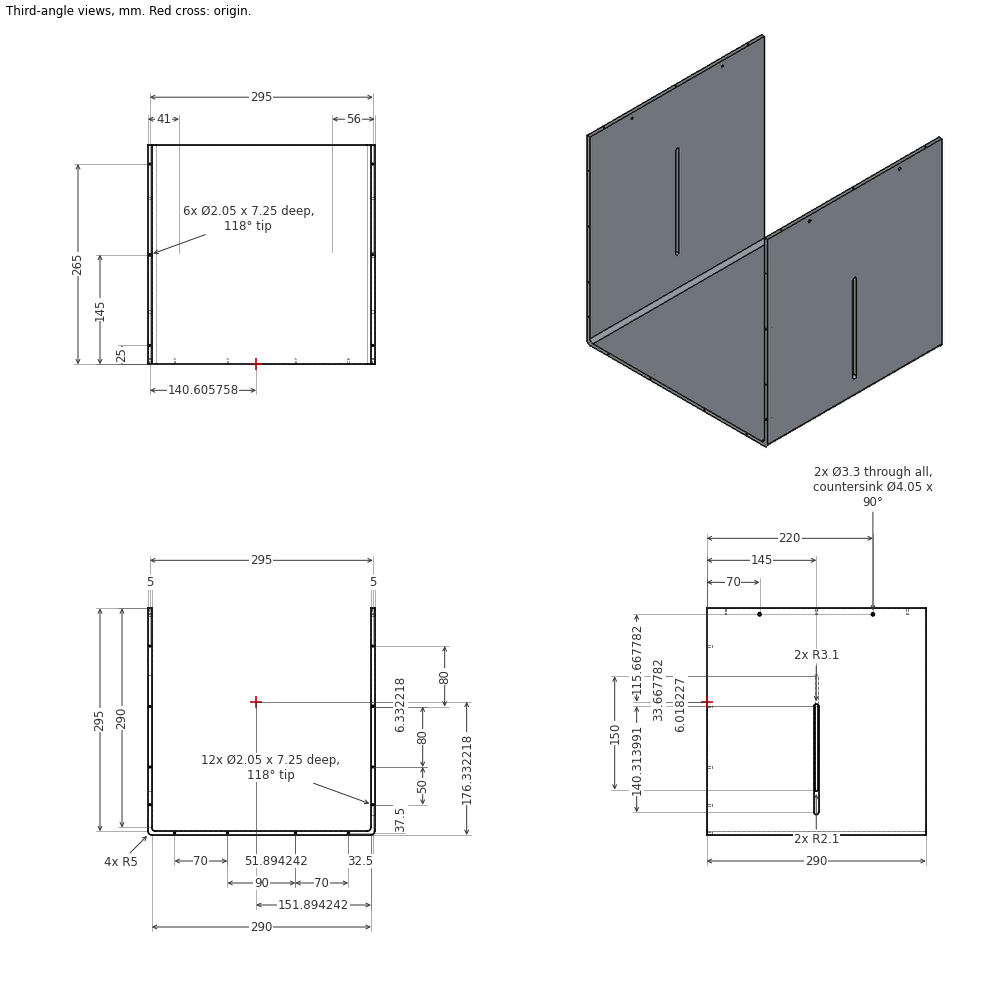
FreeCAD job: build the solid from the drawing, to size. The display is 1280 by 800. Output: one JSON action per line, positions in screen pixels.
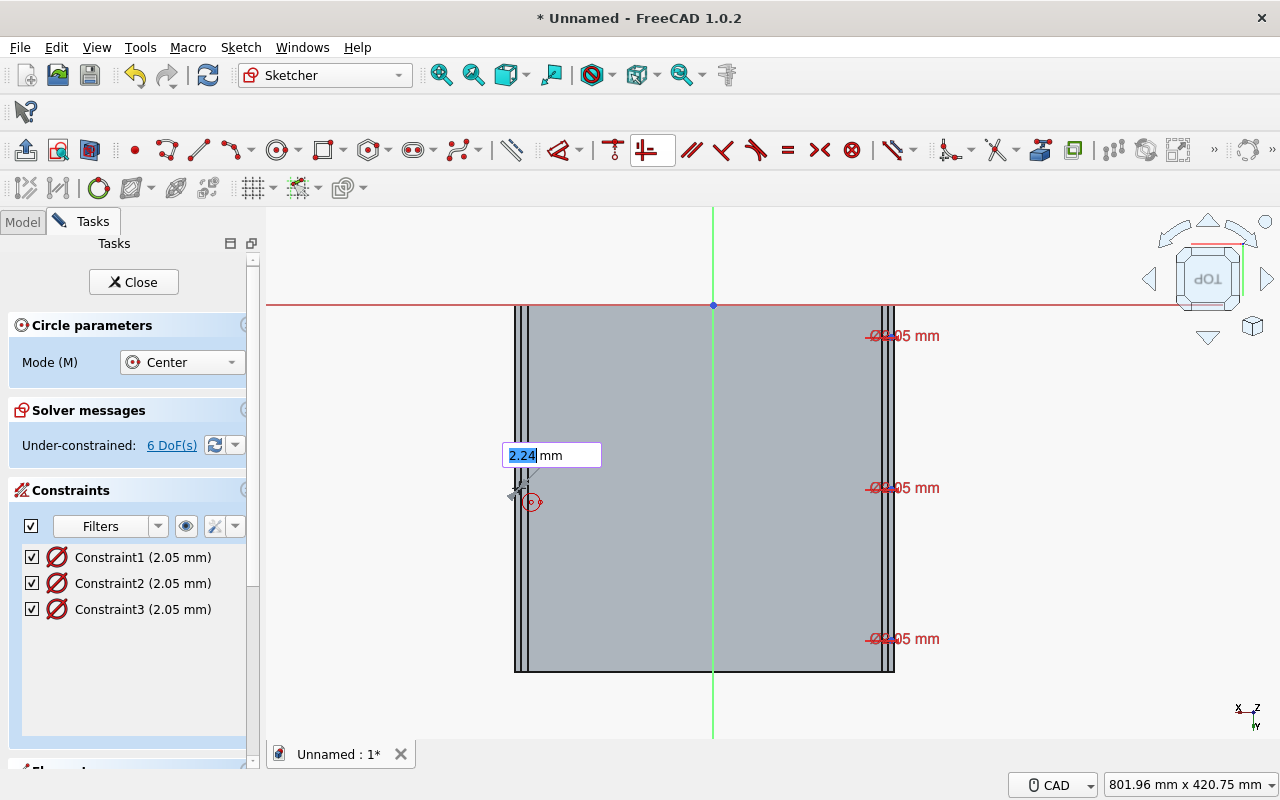
{"action": "type", "text": "2.05"}
{"action": "key", "text": "Return"}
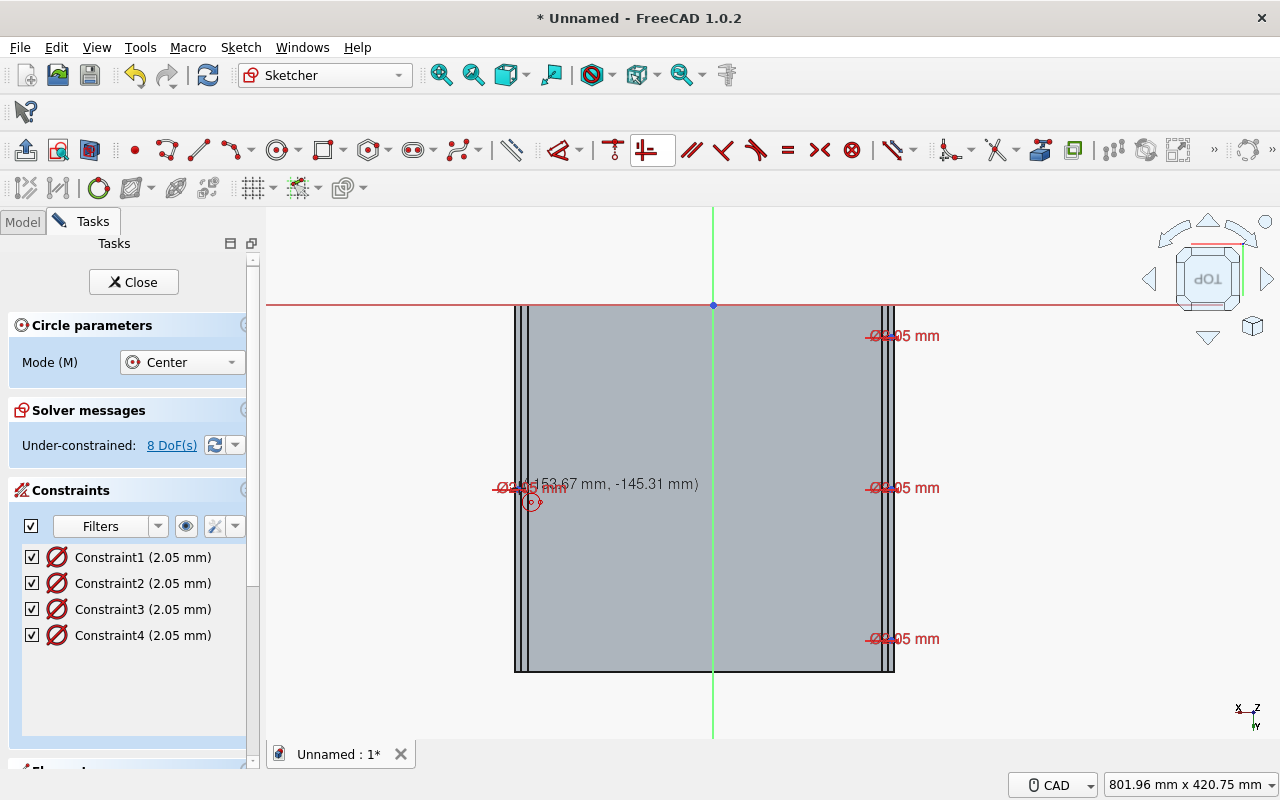
{"action": "scroll", "coordinate": [518, 640], "scroll_direction": "up", "scroll_amount": 15}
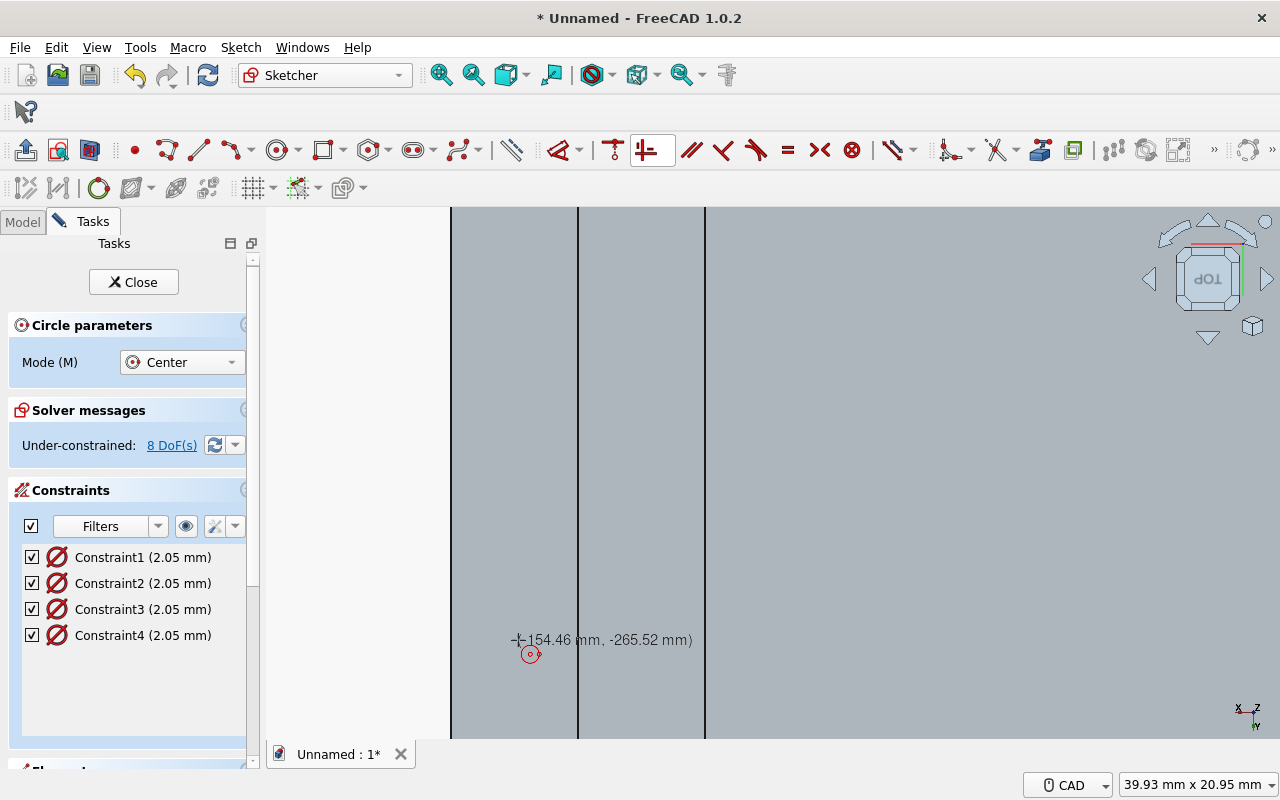
{"action": "scroll", "coordinate": [518, 640], "scroll_direction": "down", "scroll_amount": 15}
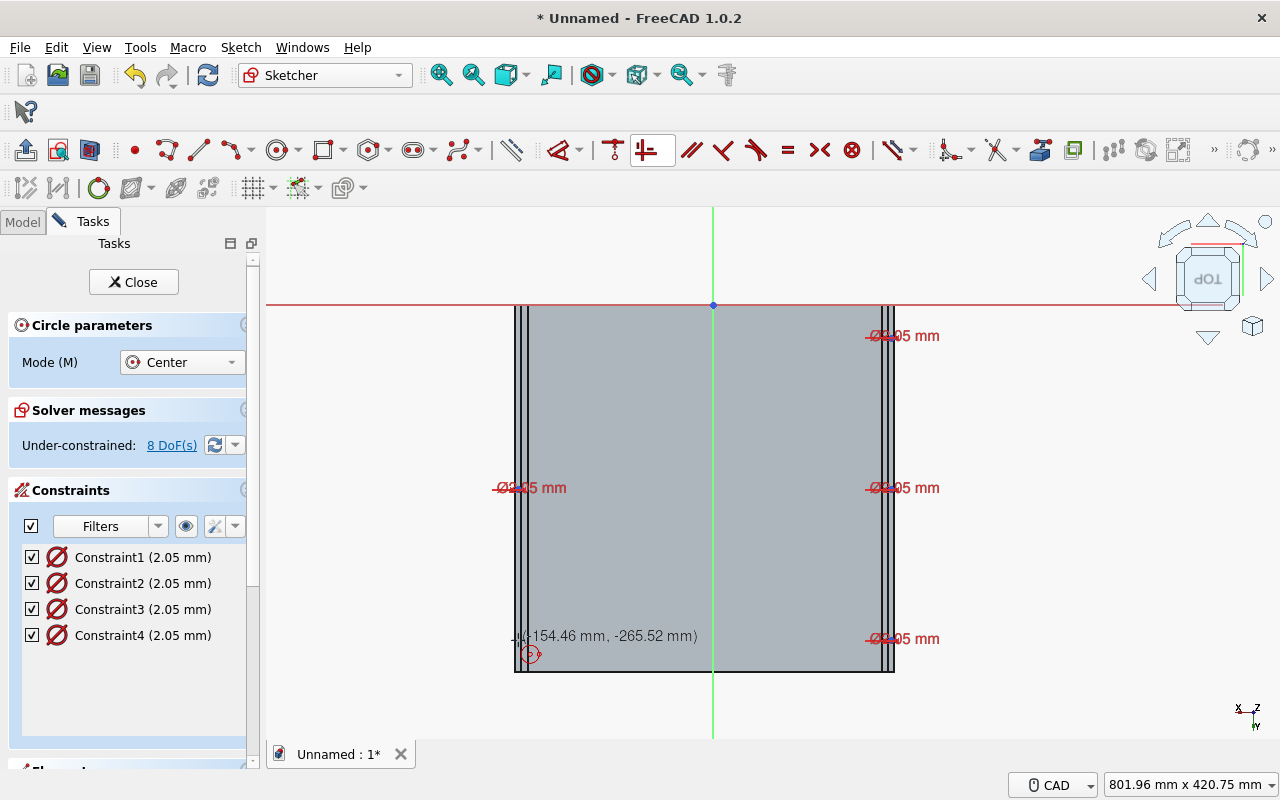
{"action": "left_click", "coordinate": [518, 640]}
{"action": "mouse_move", "coordinate": [519, 639]}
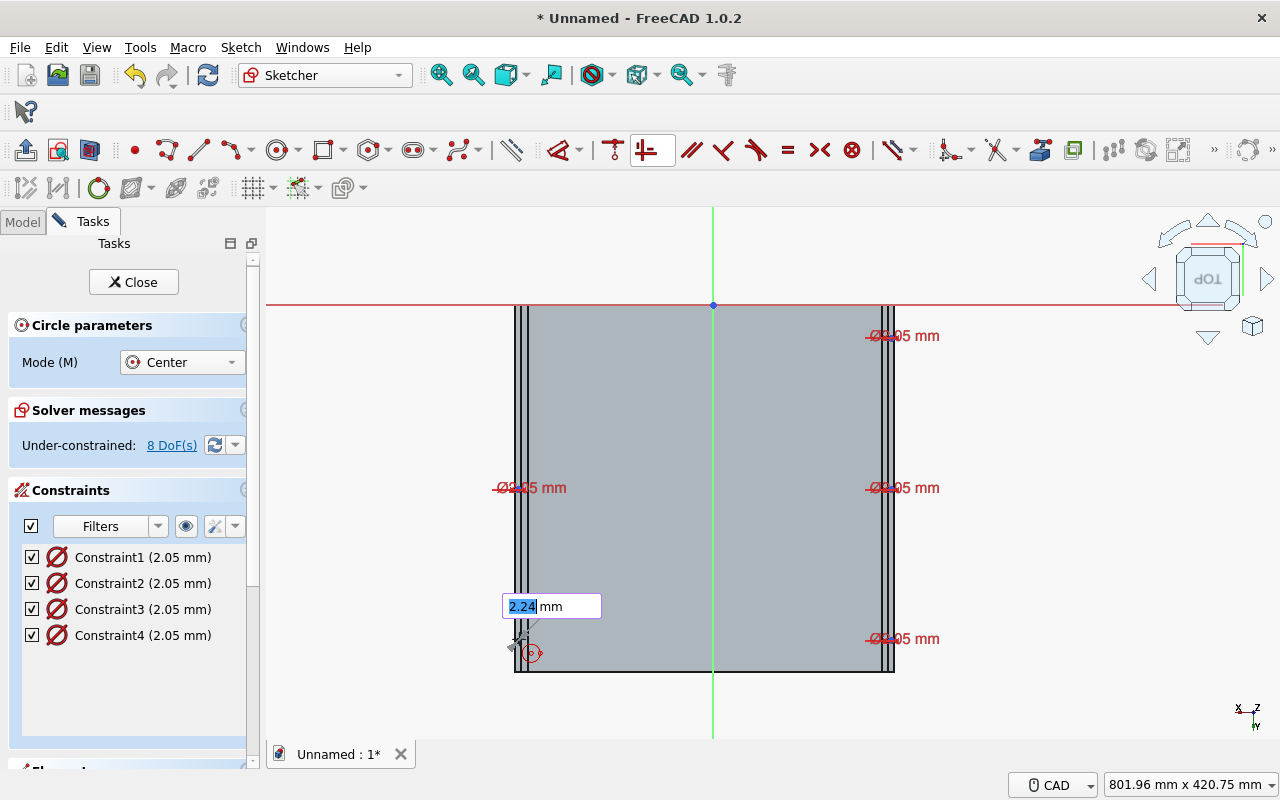
{"action": "type", "text": "2.05"}
{"action": "key", "text": "Return"}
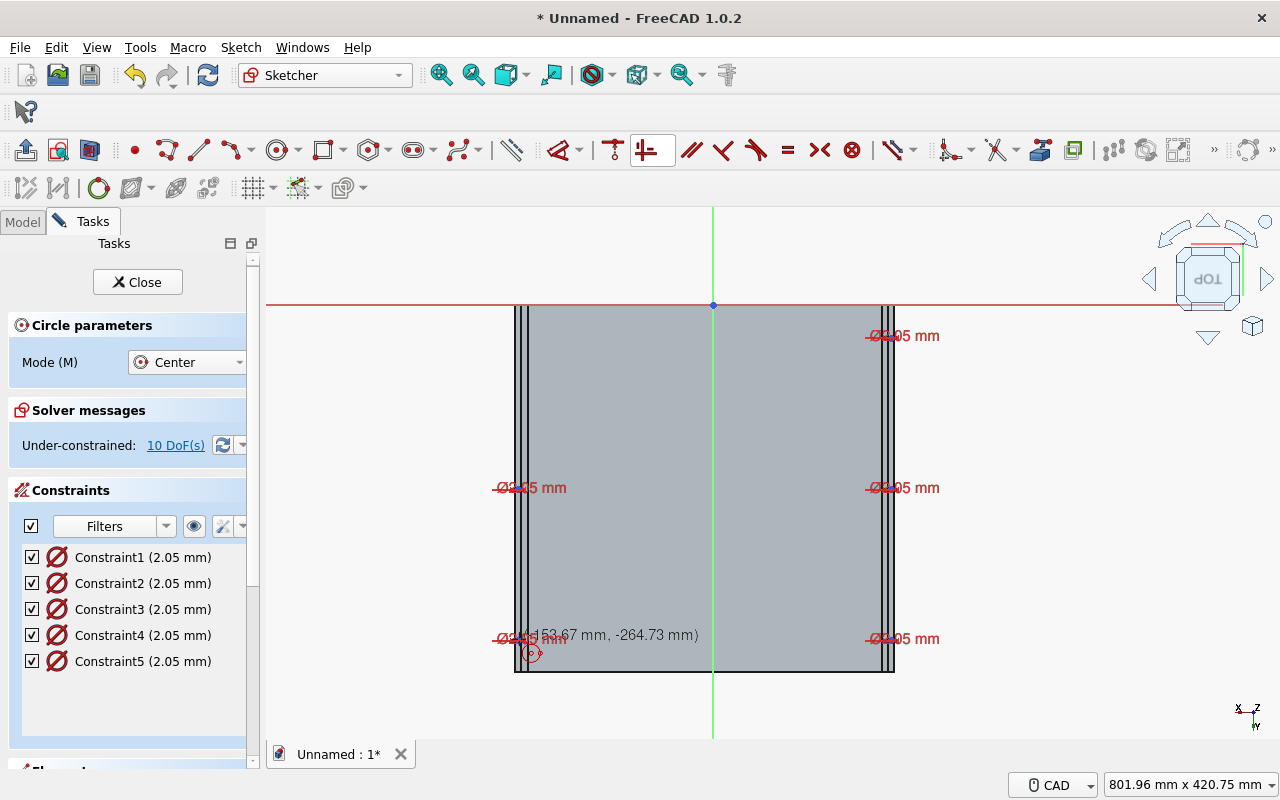
{"action": "scroll", "coordinate": [518, 337], "scroll_direction": "up", "scroll_amount": 15}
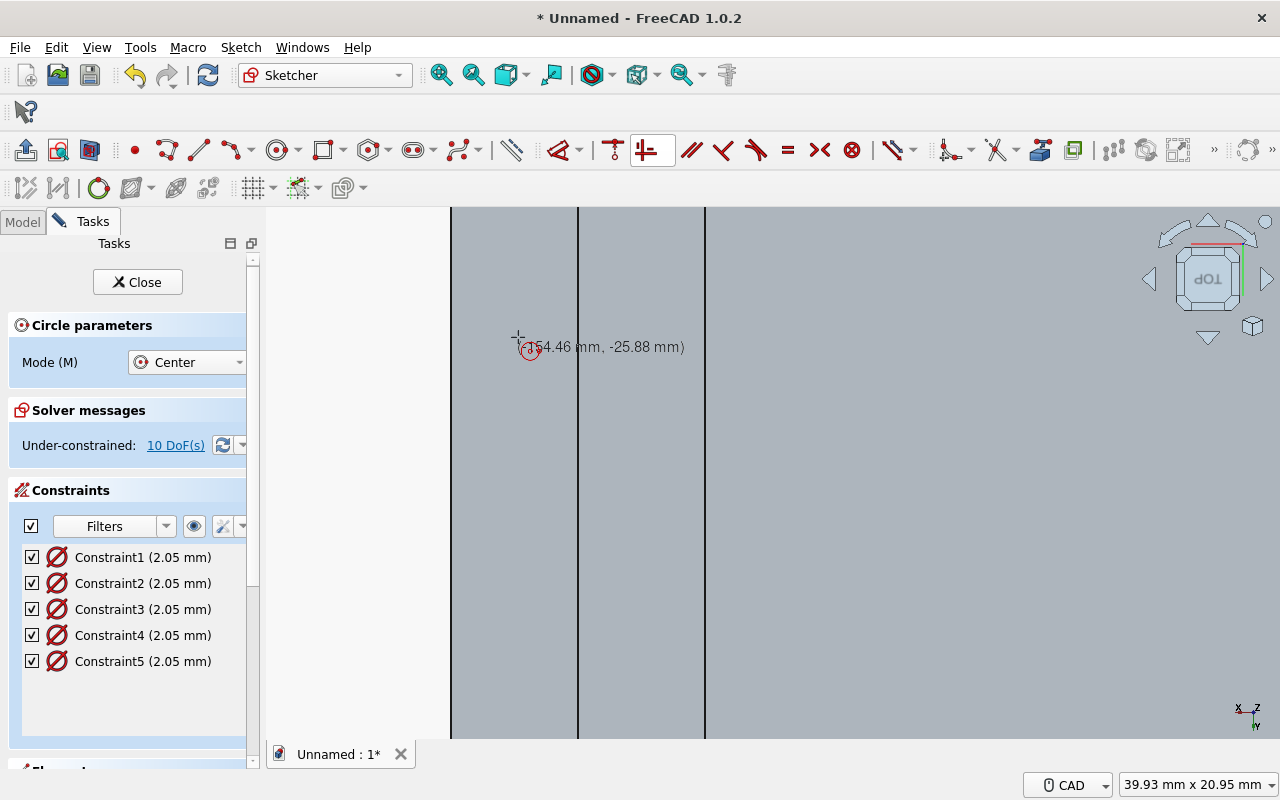
{"action": "scroll", "coordinate": [518, 337], "scroll_direction": "down", "scroll_amount": 15}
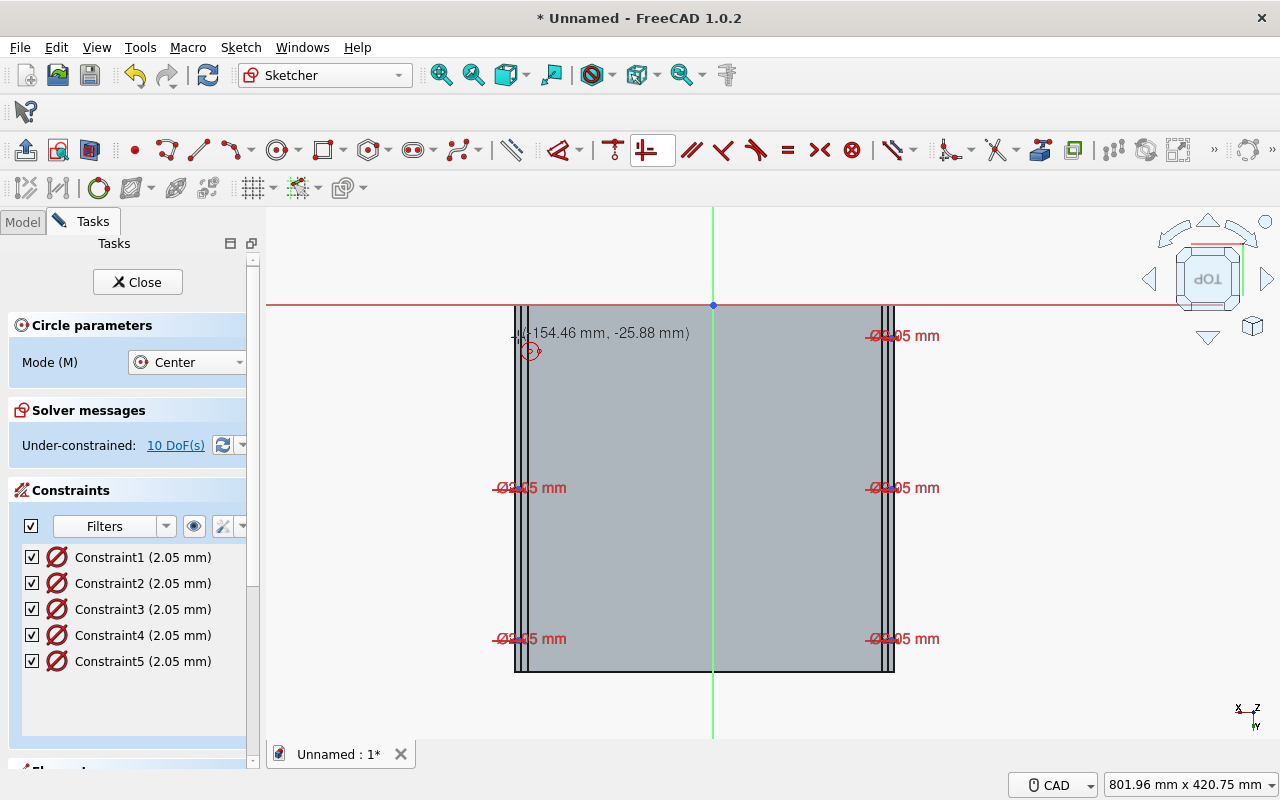
{"action": "left_click", "coordinate": [518, 337]}
{"action": "mouse_move", "coordinate": [519, 336]}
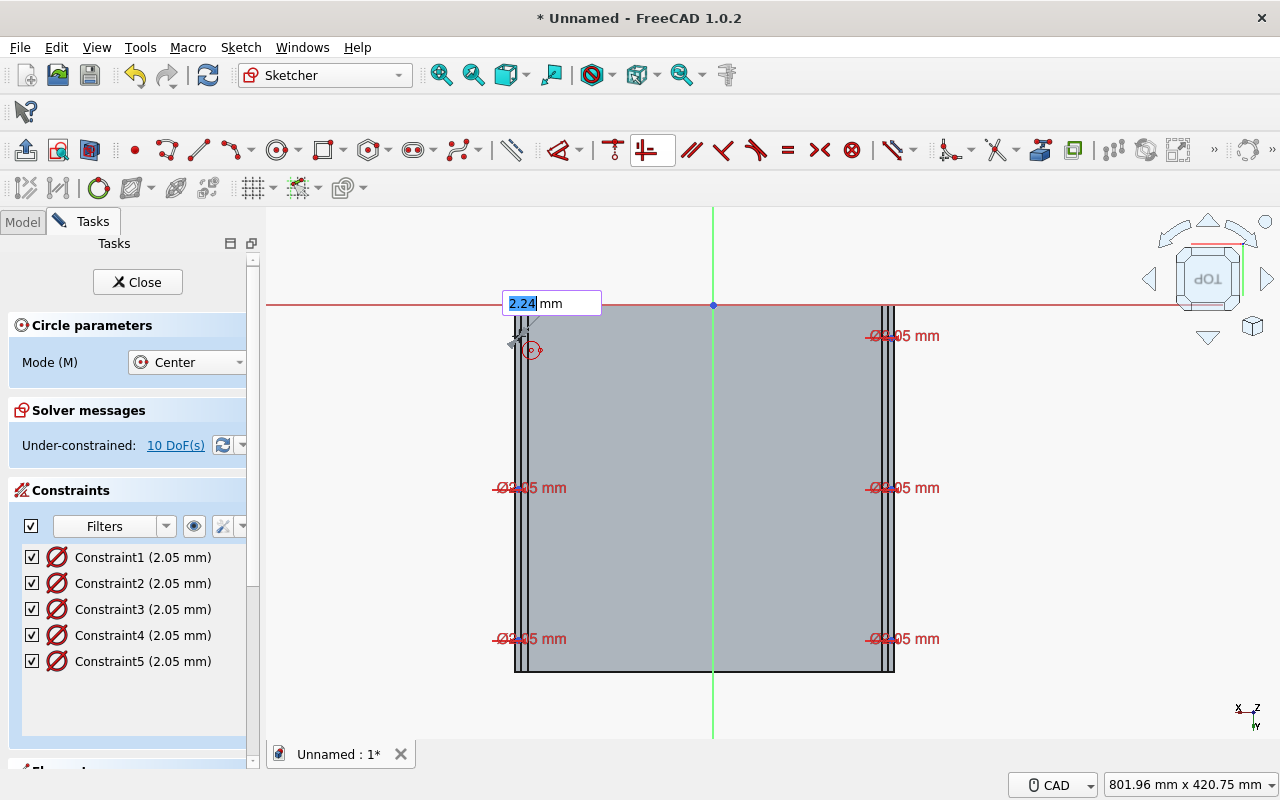
{"action": "type", "text": "2.05"}
{"action": "key", "text": "Return"}
{"action": "key", "text": "Escape"}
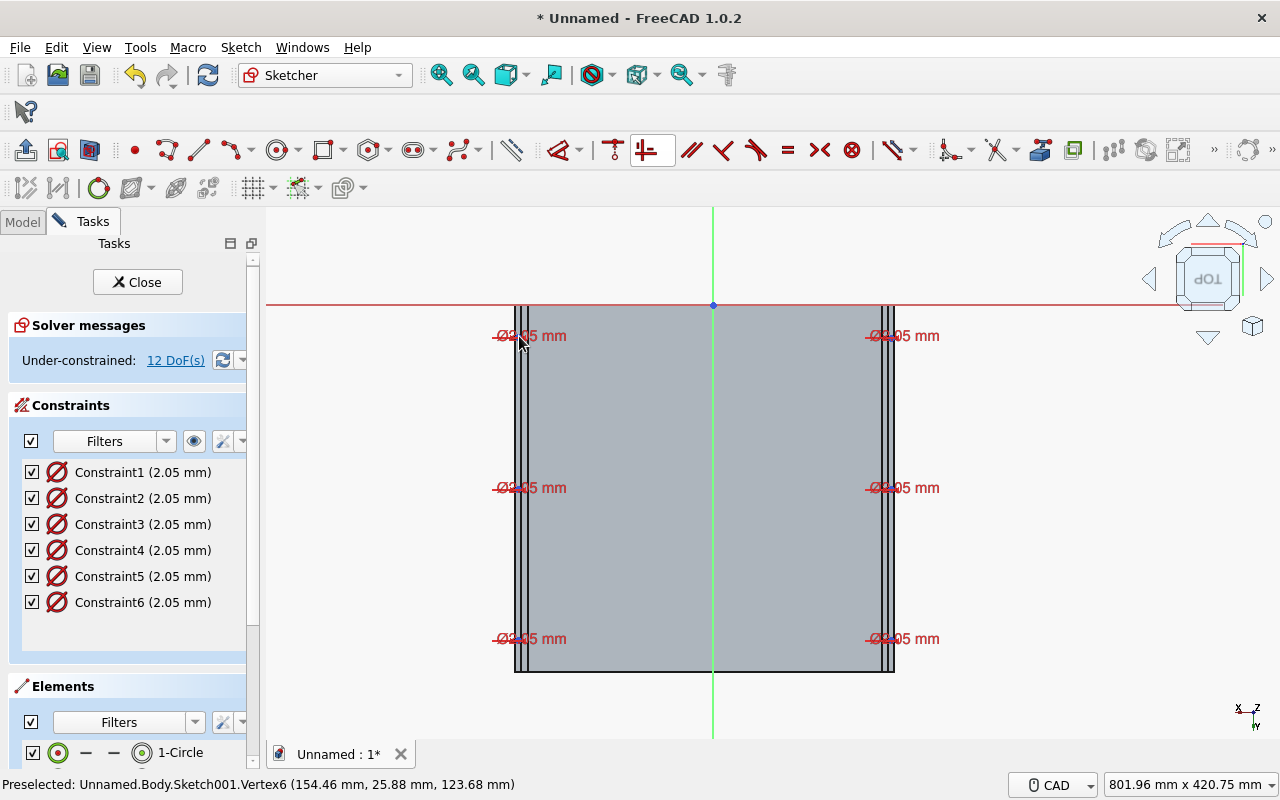
{"action": "left_click", "coordinate": [891, 490]}